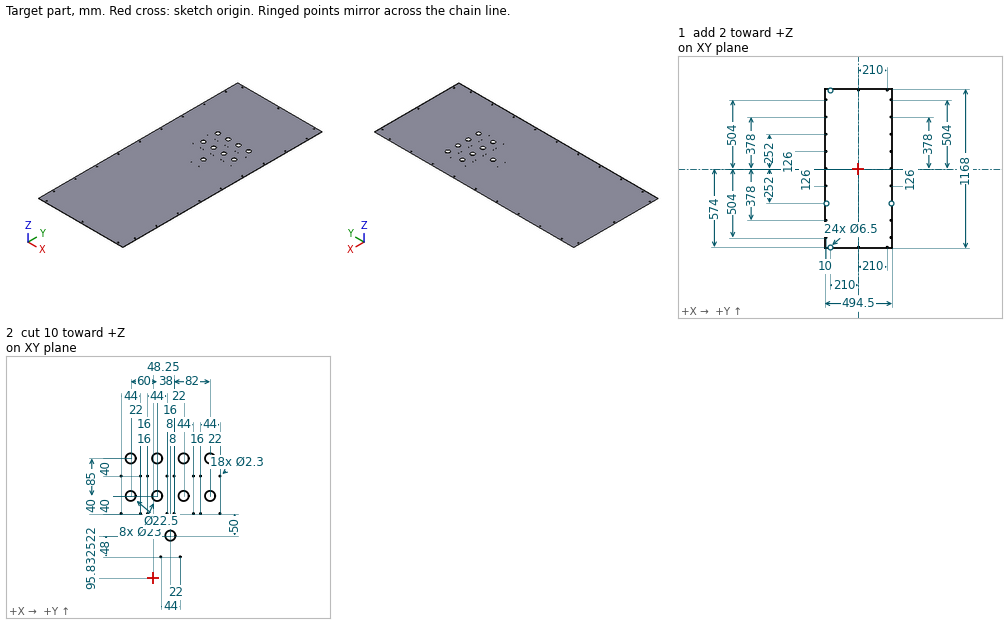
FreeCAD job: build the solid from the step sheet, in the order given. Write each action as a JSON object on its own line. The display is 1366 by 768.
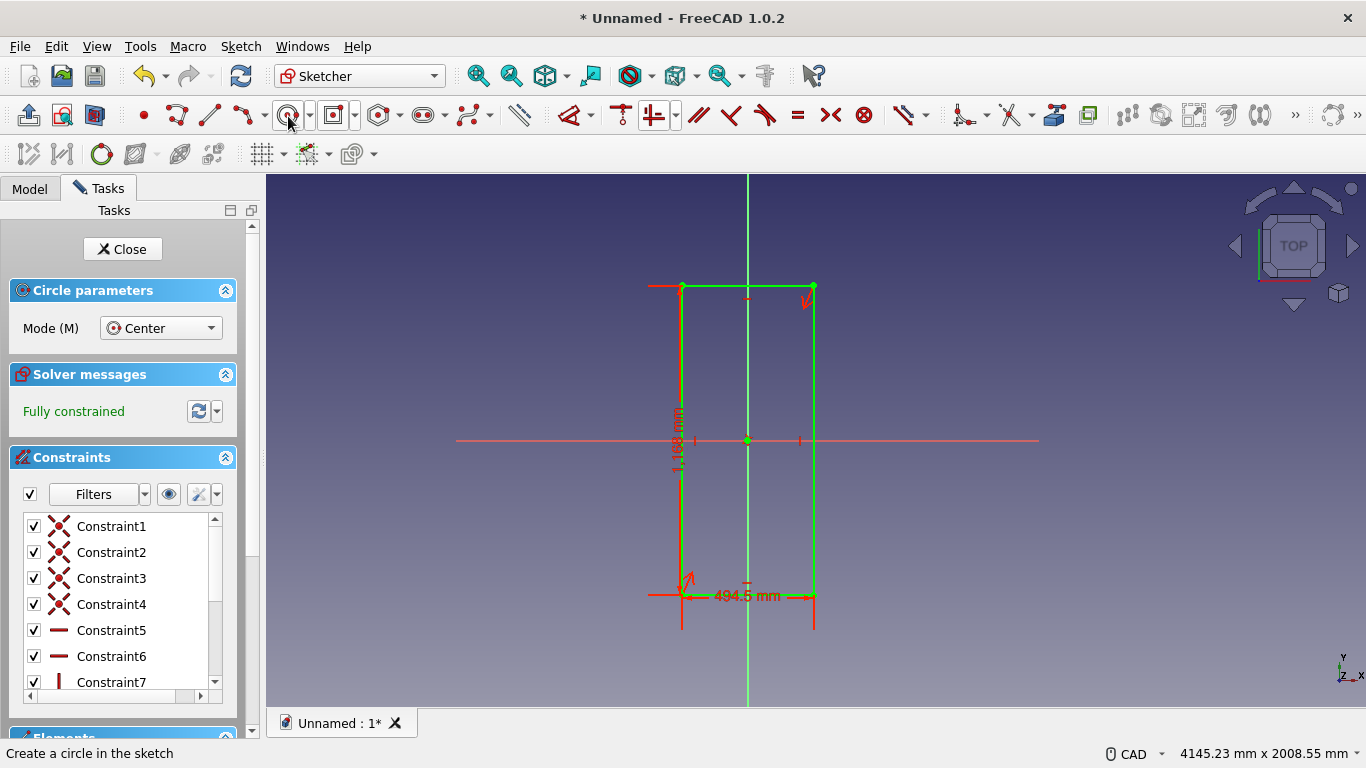
{"action": "scroll", "coordinate": [692, 593], "scroll_direction": "up", "scroll_amount": 17}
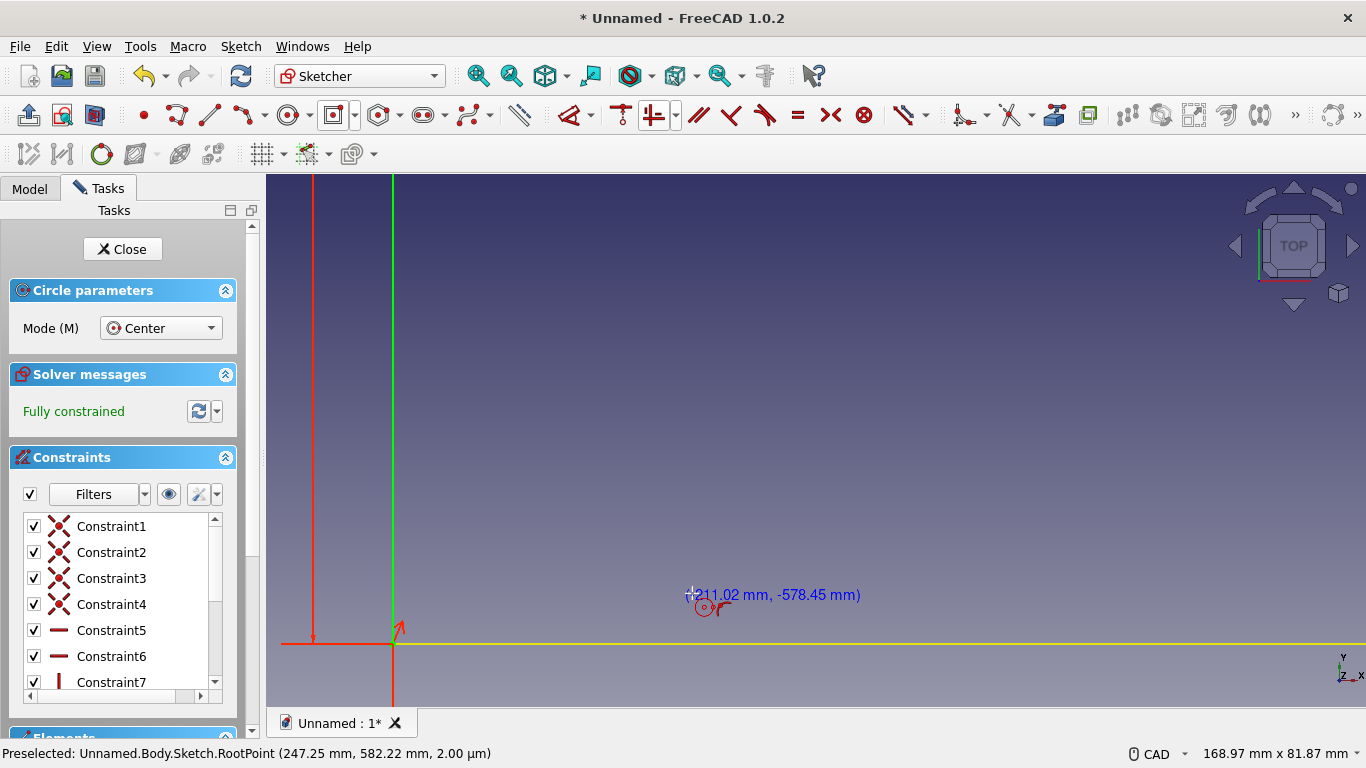
{"action": "scroll", "coordinate": [679, 629], "scroll_direction": "down", "scroll_amount": 16}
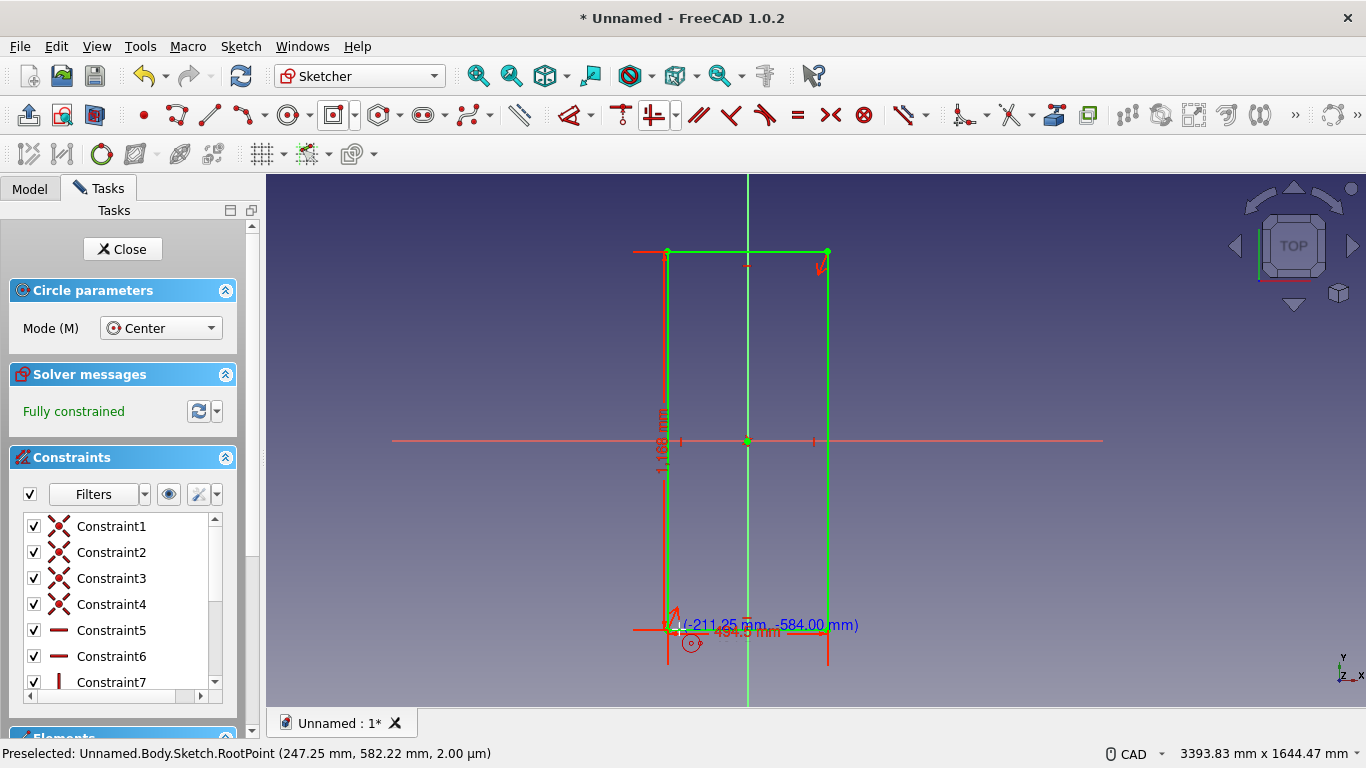
{"action": "scroll", "coordinate": [680, 627], "scroll_direction": "up", "scroll_amount": 8}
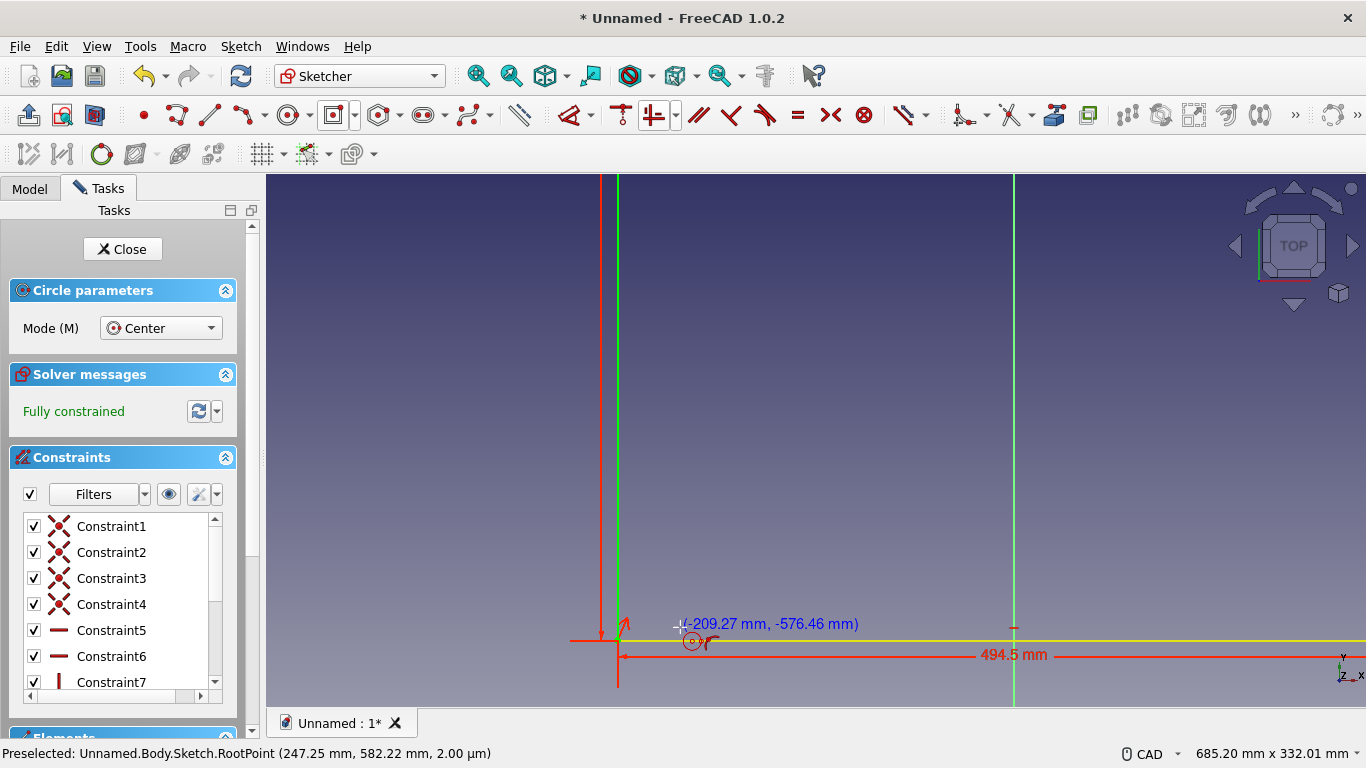
{"action": "left_click", "coordinate": [677, 625]}
{"action": "mouse_move", "coordinate": [681, 621]}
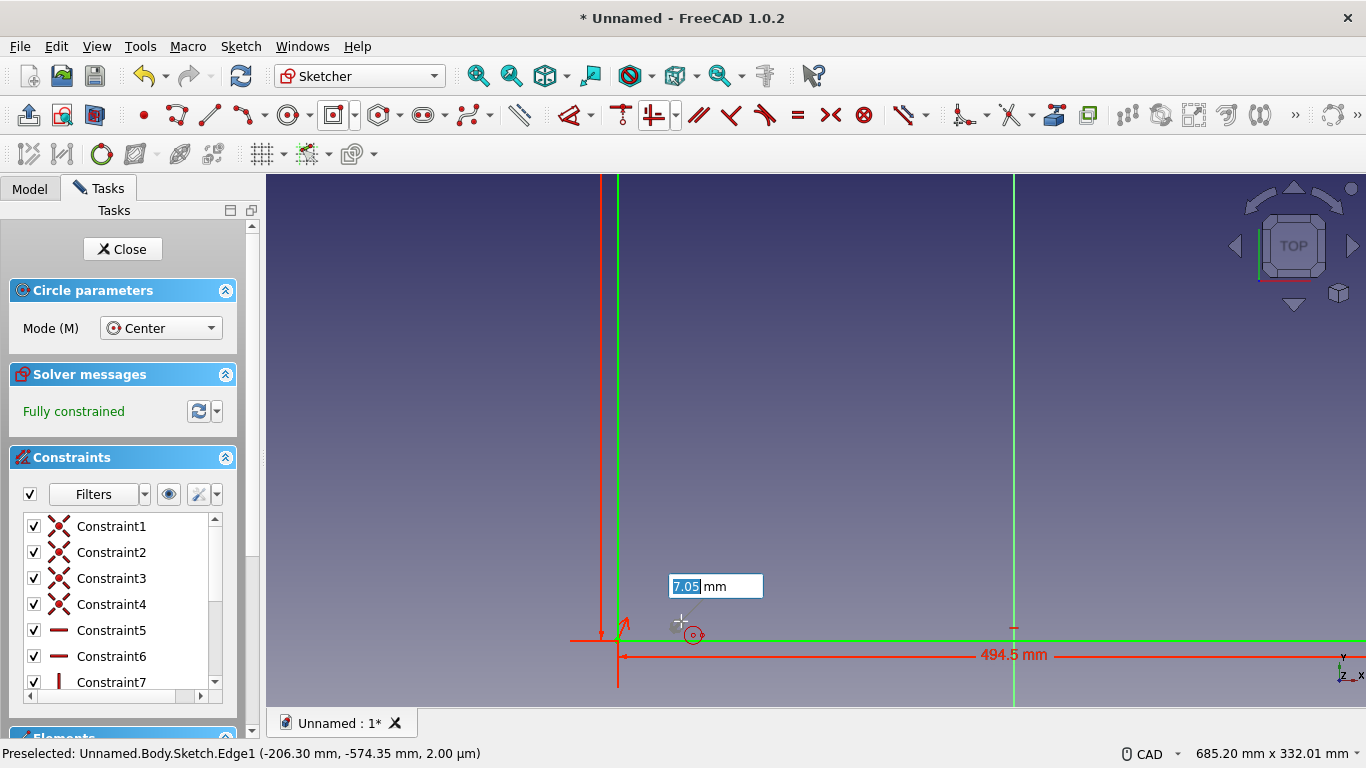
{"action": "type", "text": "6.5"}
{"action": "key", "text": "Return"}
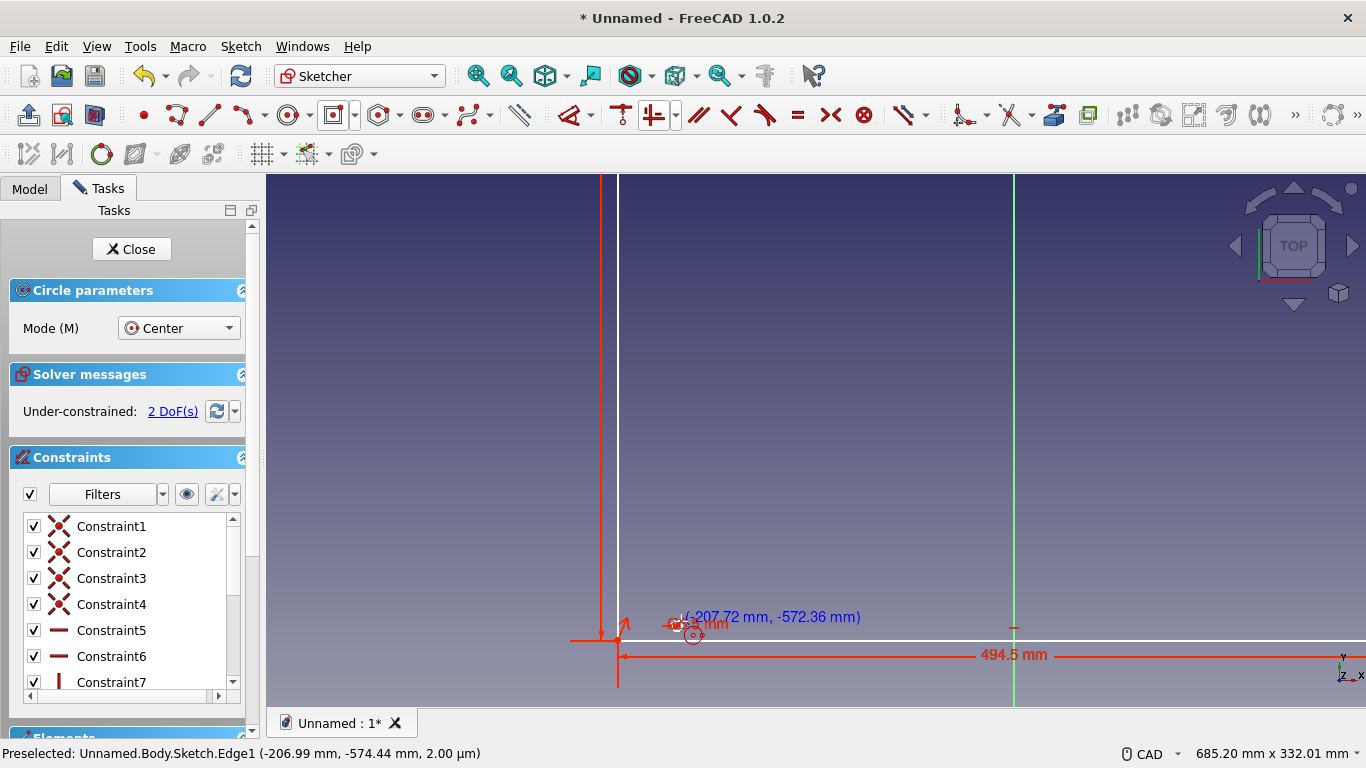
{"action": "scroll", "coordinate": [634, 512], "scroll_direction": "up", "scroll_amount": 8}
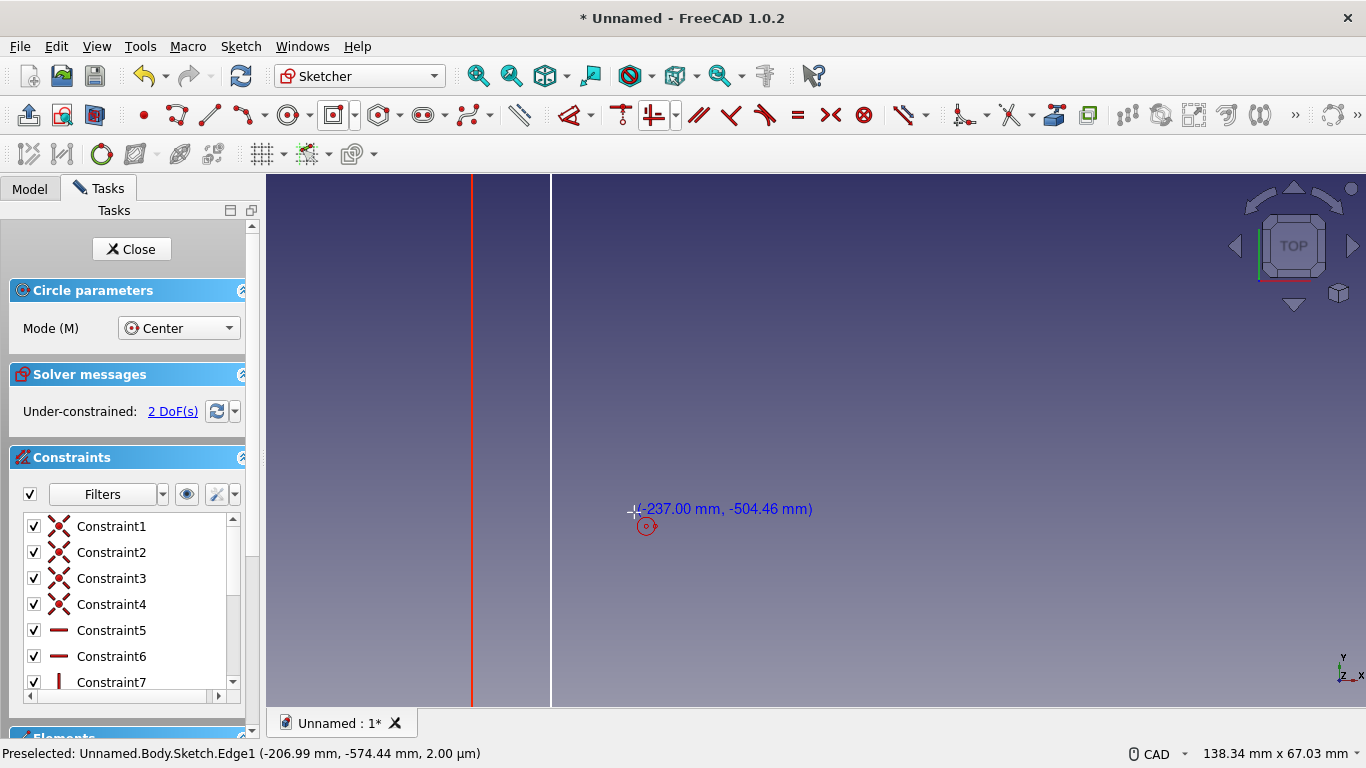
{"action": "scroll", "coordinate": [672, 608], "scroll_direction": "down", "scroll_amount": 16}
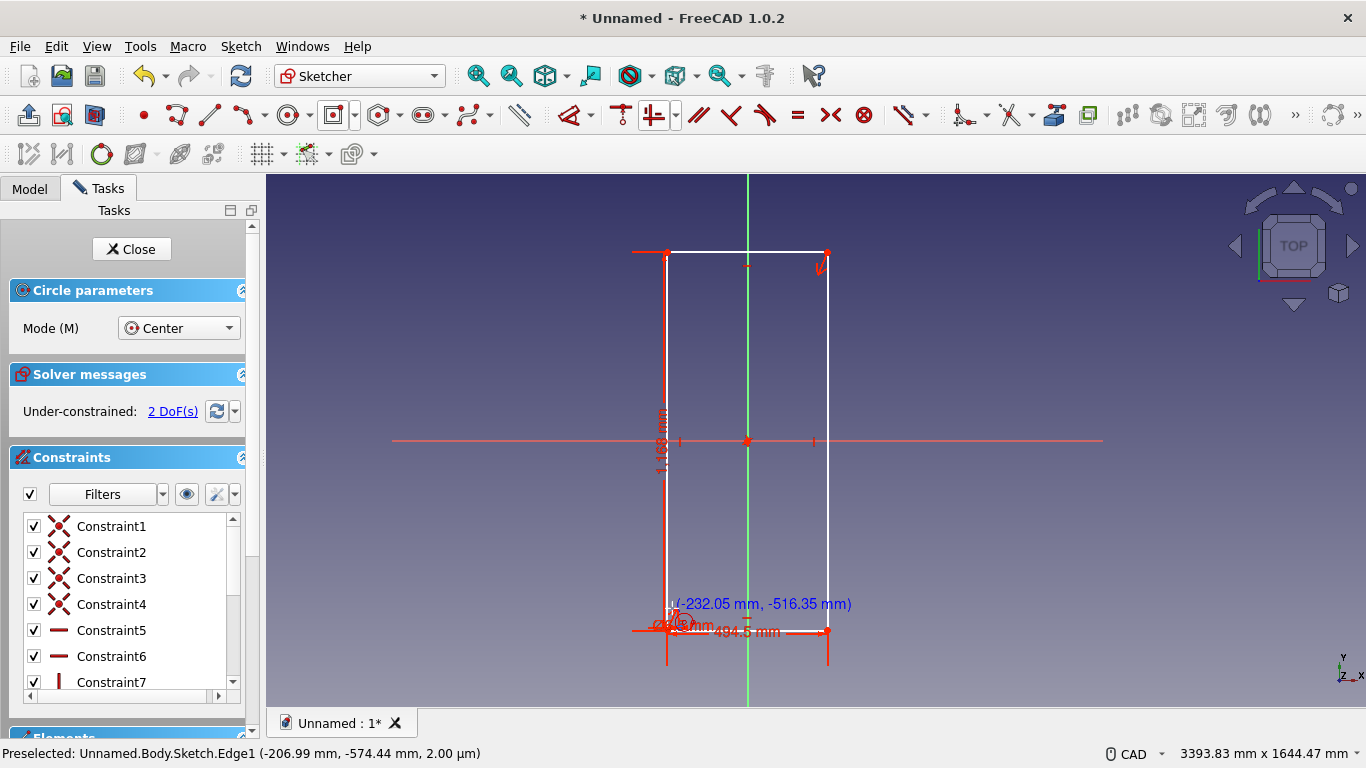
{"action": "scroll", "coordinate": [671, 605], "scroll_direction": "up", "scroll_amount": 8}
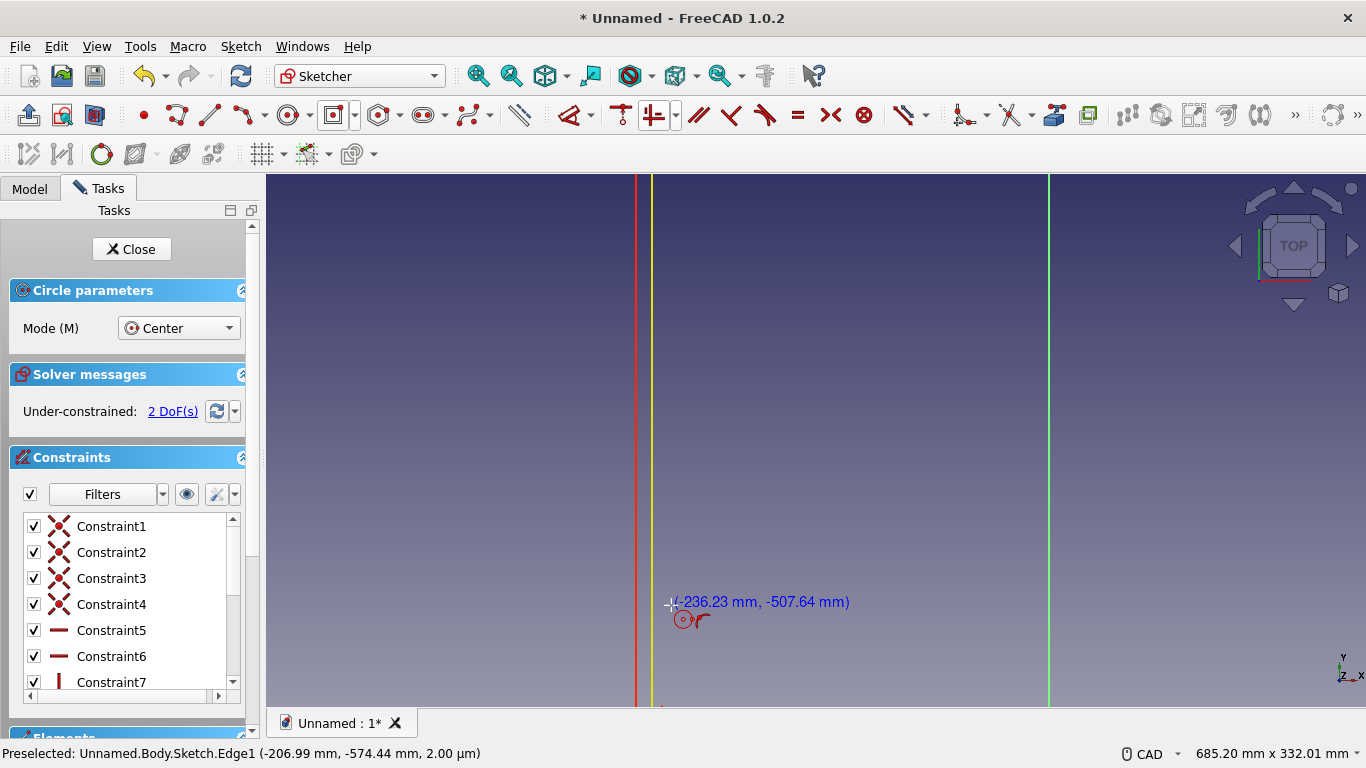
{"action": "left_click", "coordinate": [668, 601]}
{"action": "mouse_move", "coordinate": [672, 597]}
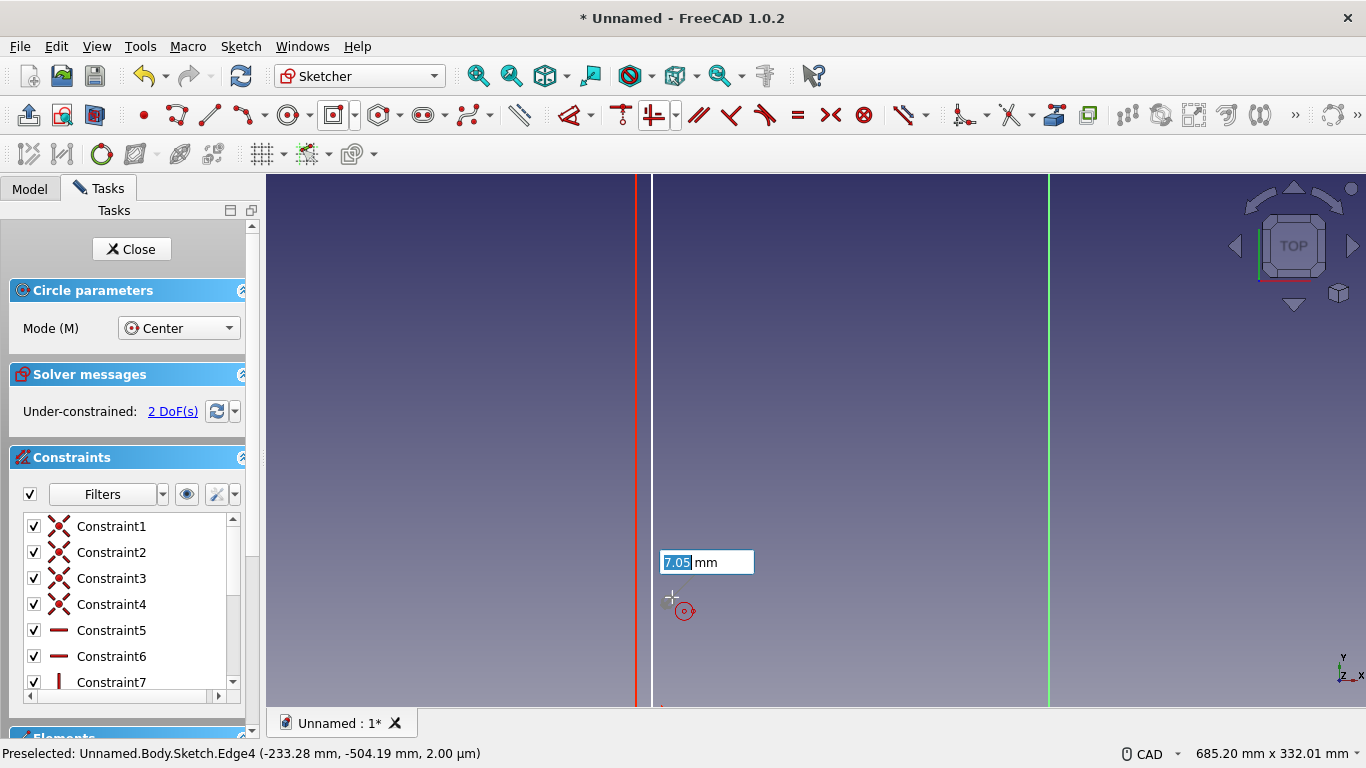
{"action": "type", "text": "6.5"}
{"action": "key", "text": "Return"}